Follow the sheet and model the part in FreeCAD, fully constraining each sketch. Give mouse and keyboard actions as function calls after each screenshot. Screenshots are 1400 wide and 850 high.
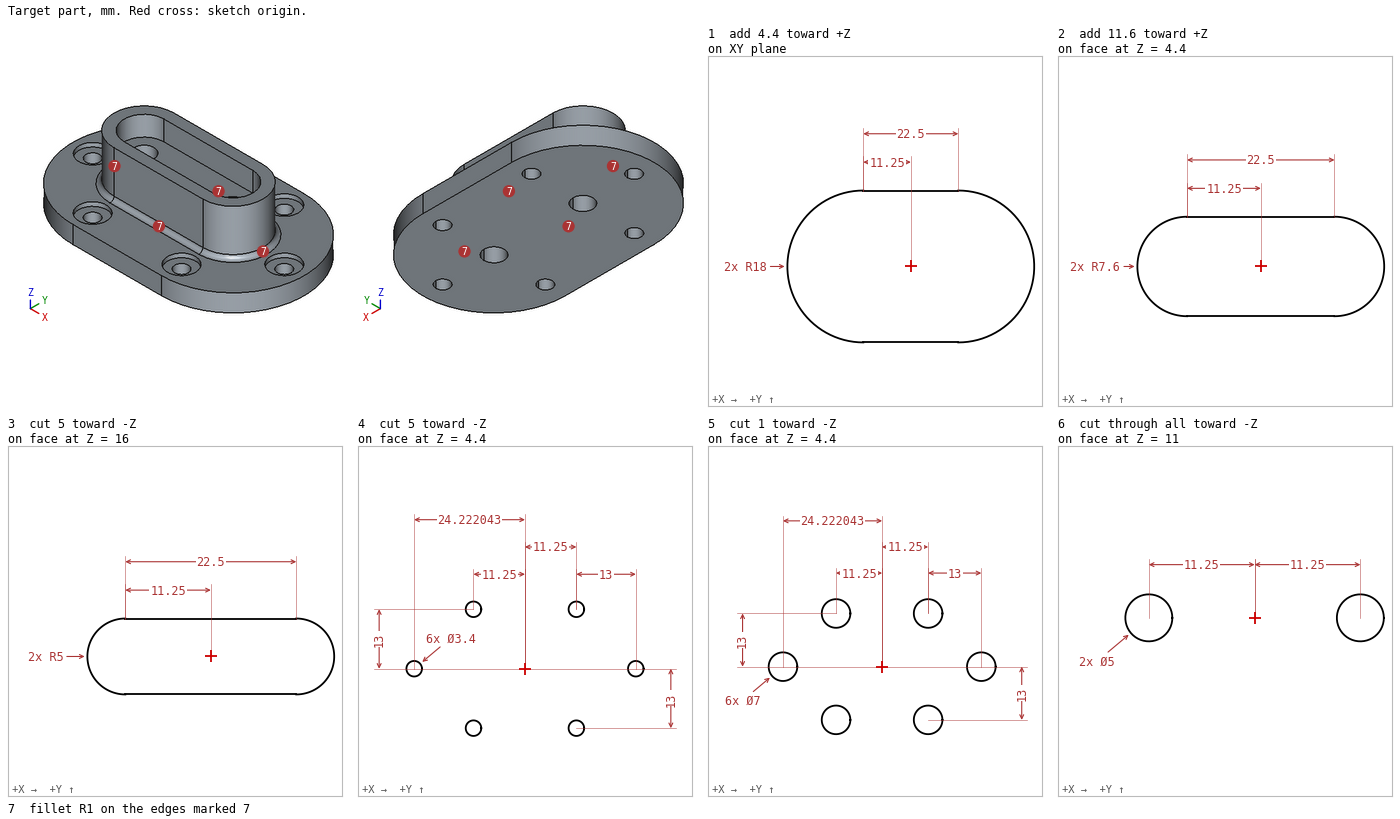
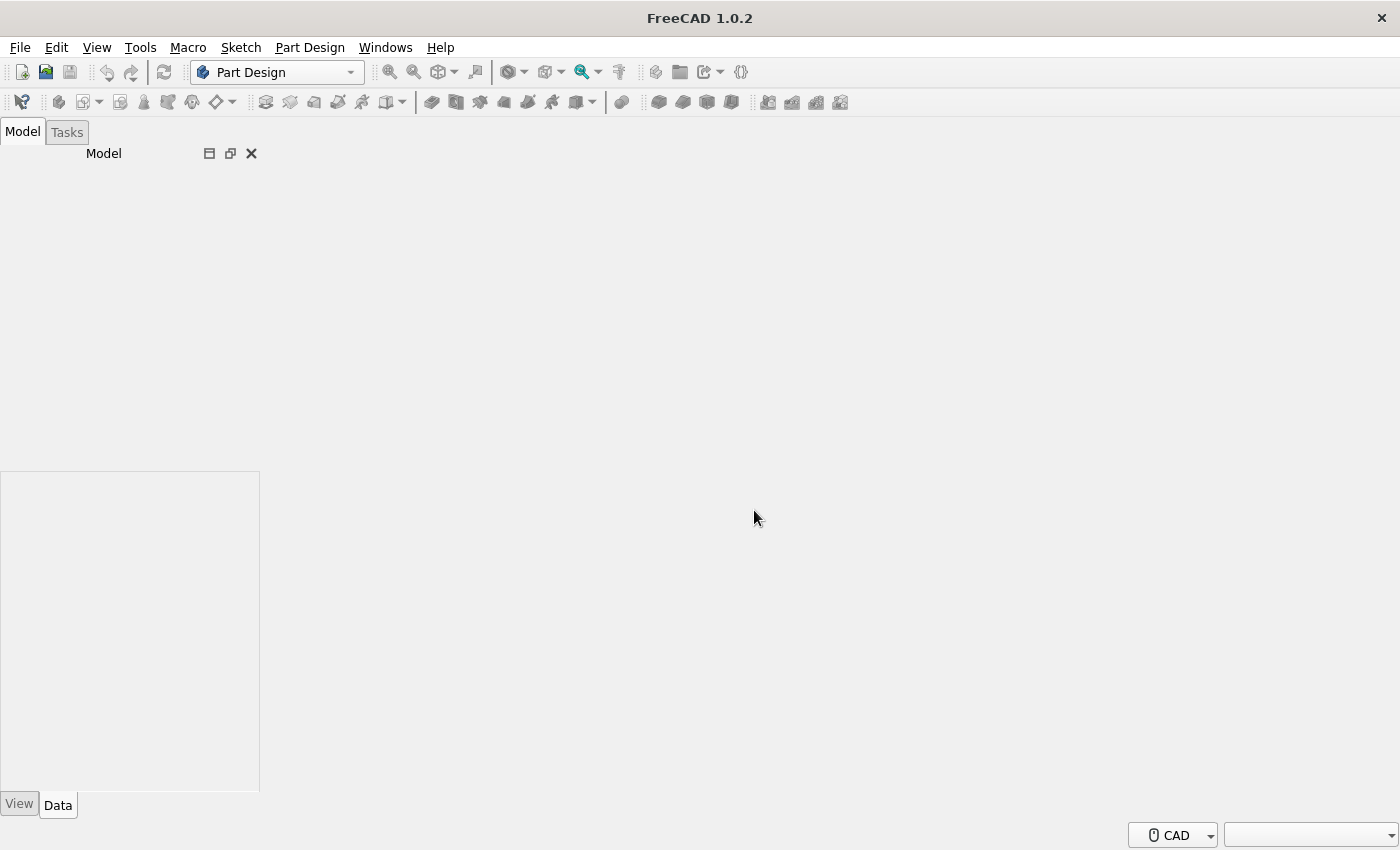
click(22, 72)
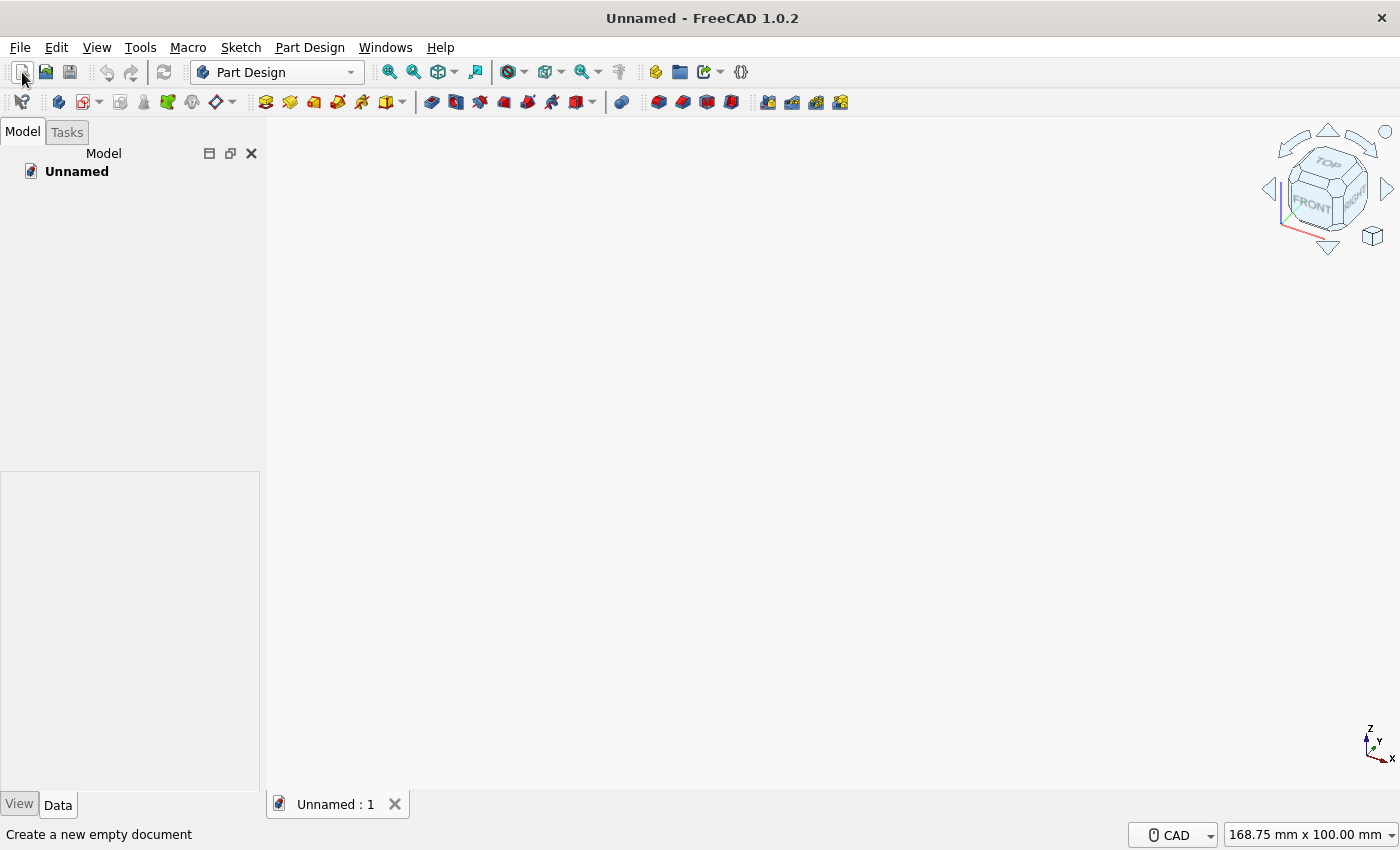
click(84, 102)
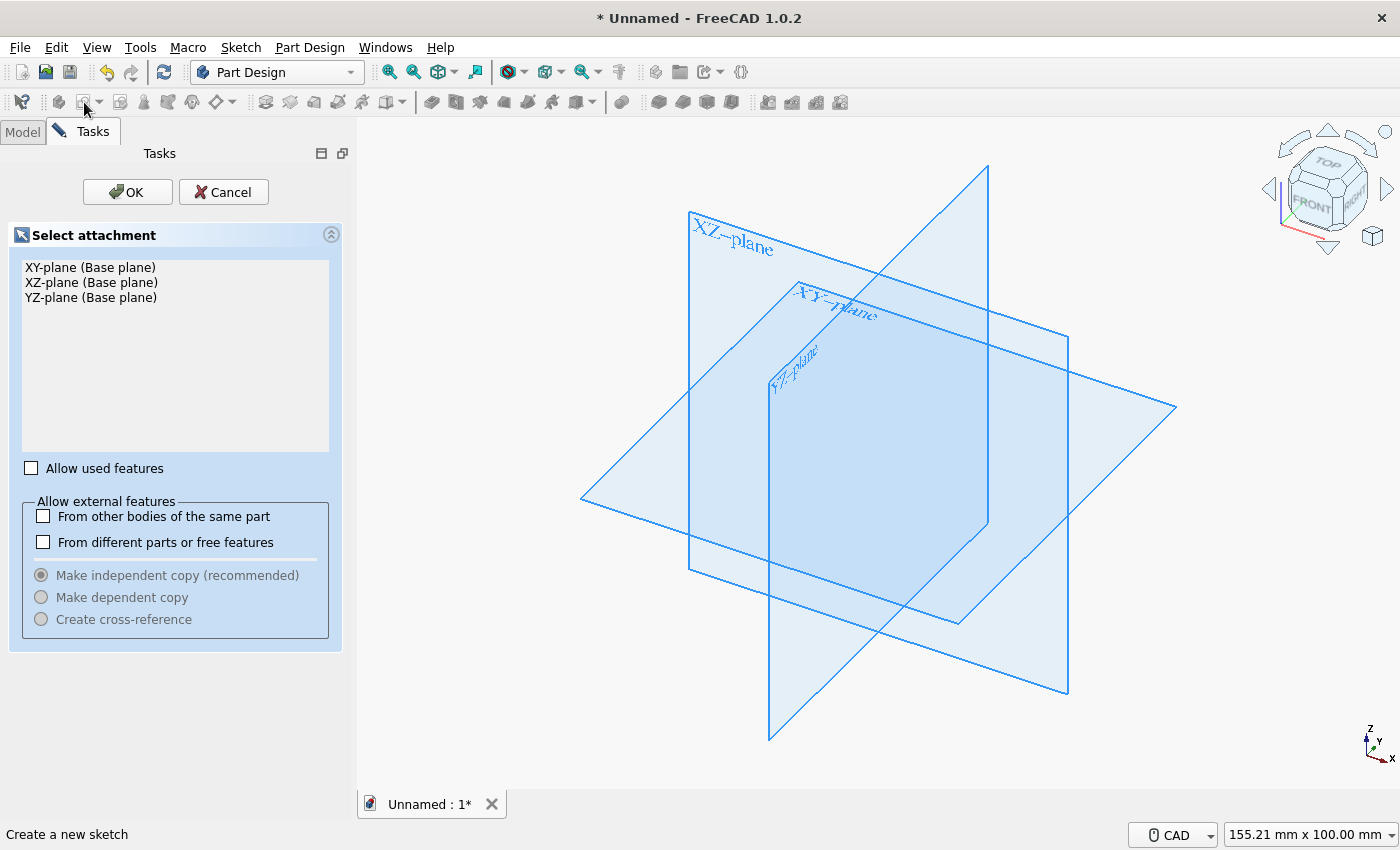
click(82, 268)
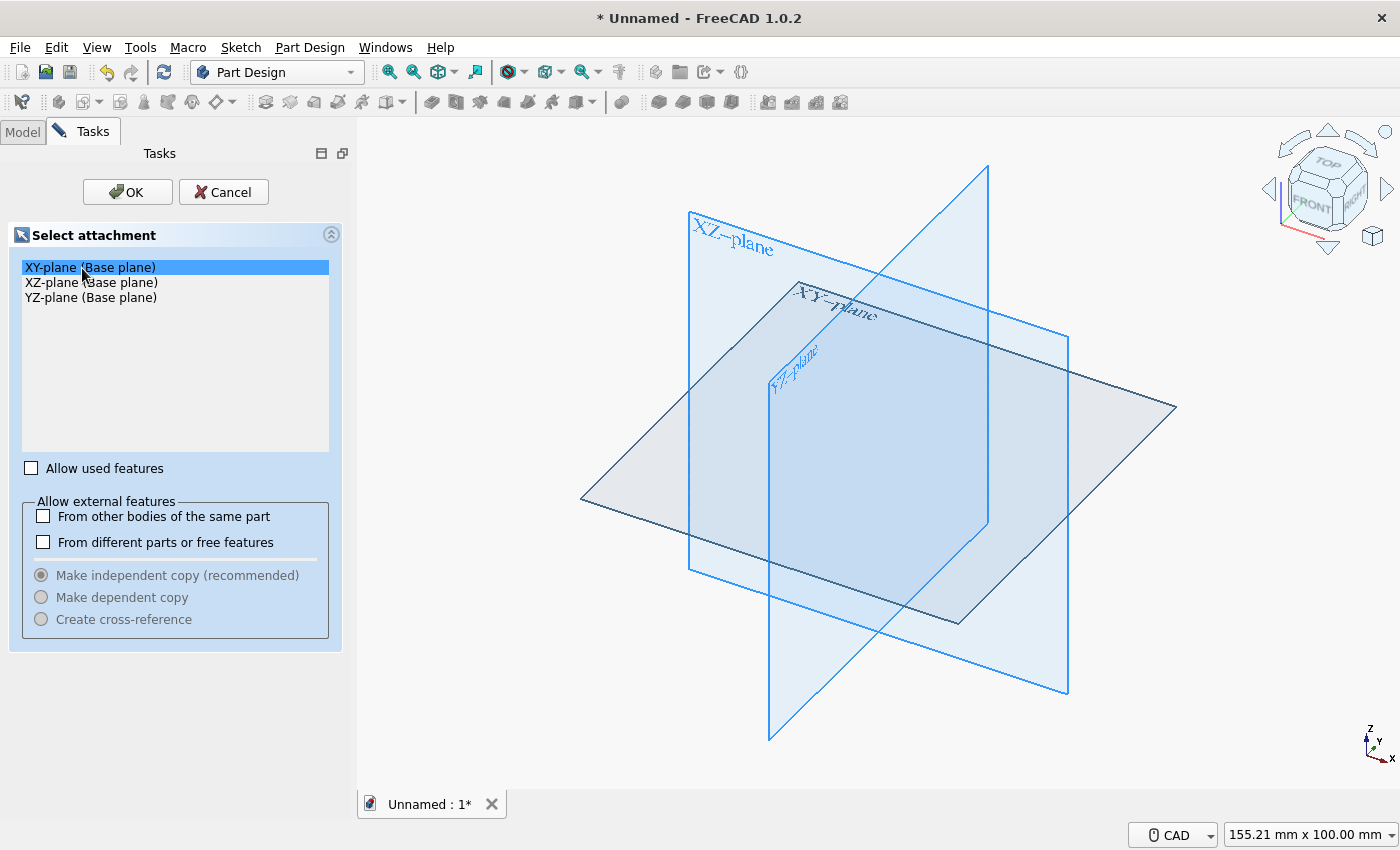
click(128, 192)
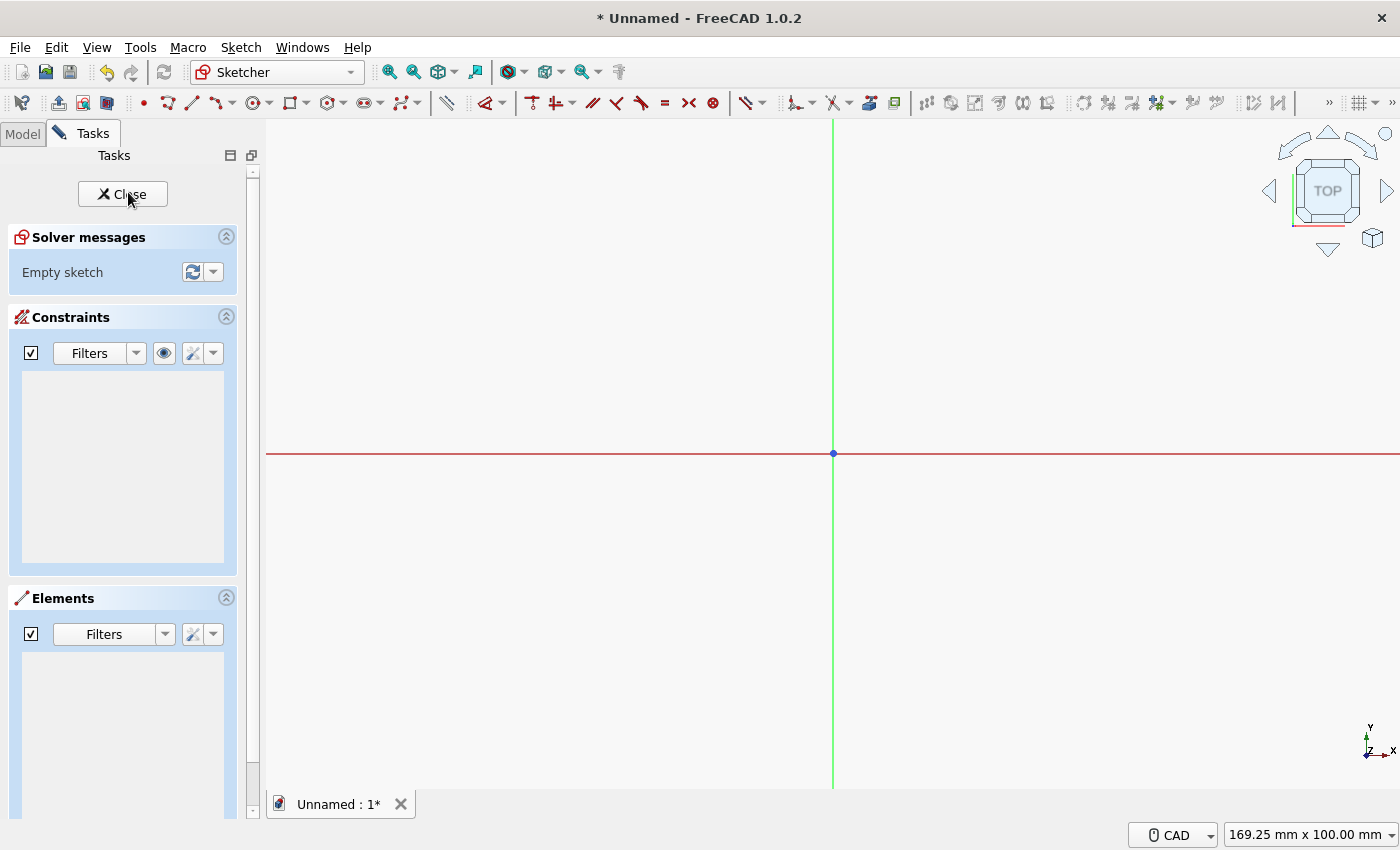
scroll(916, 454, up, 3)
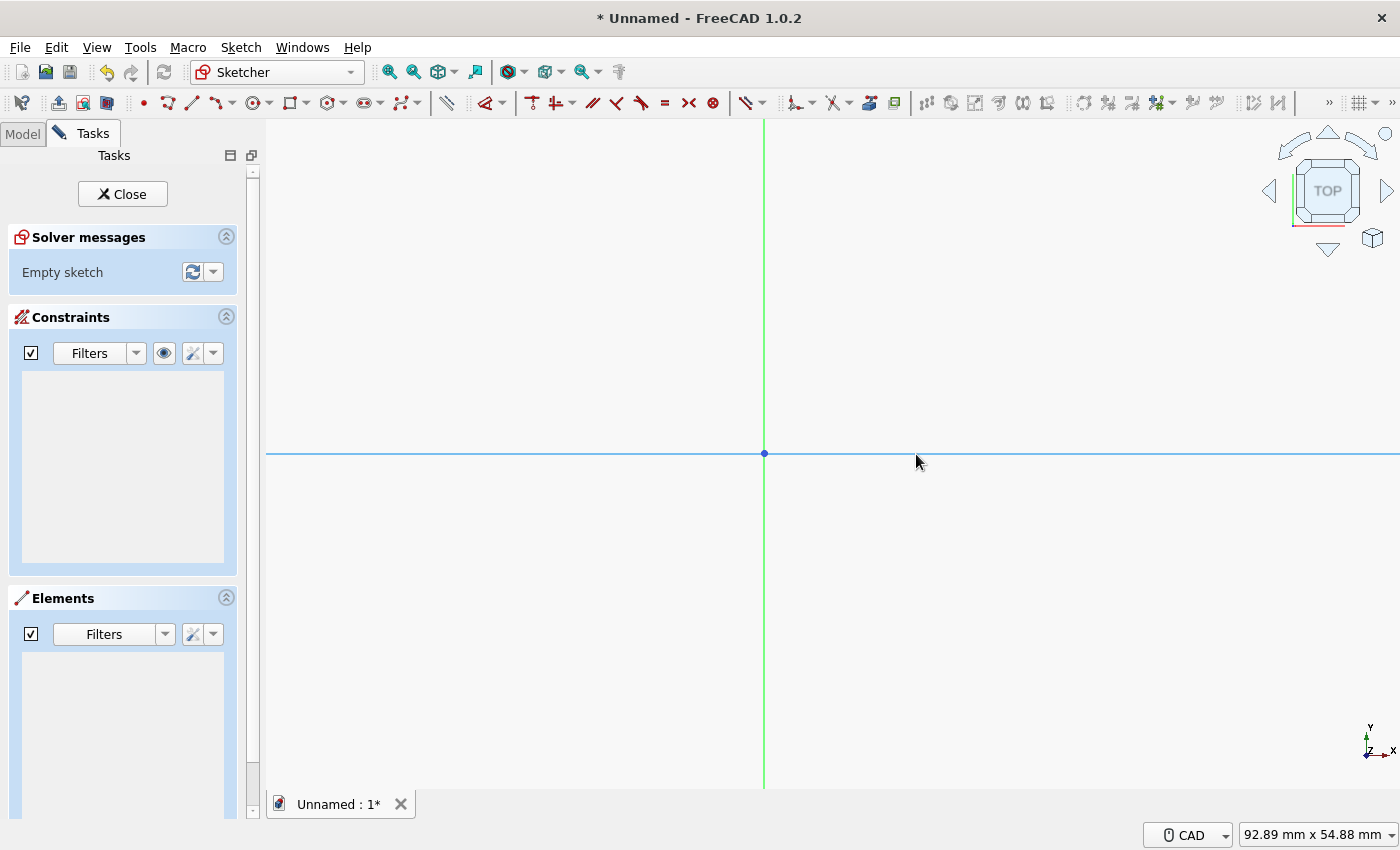
click(364, 104)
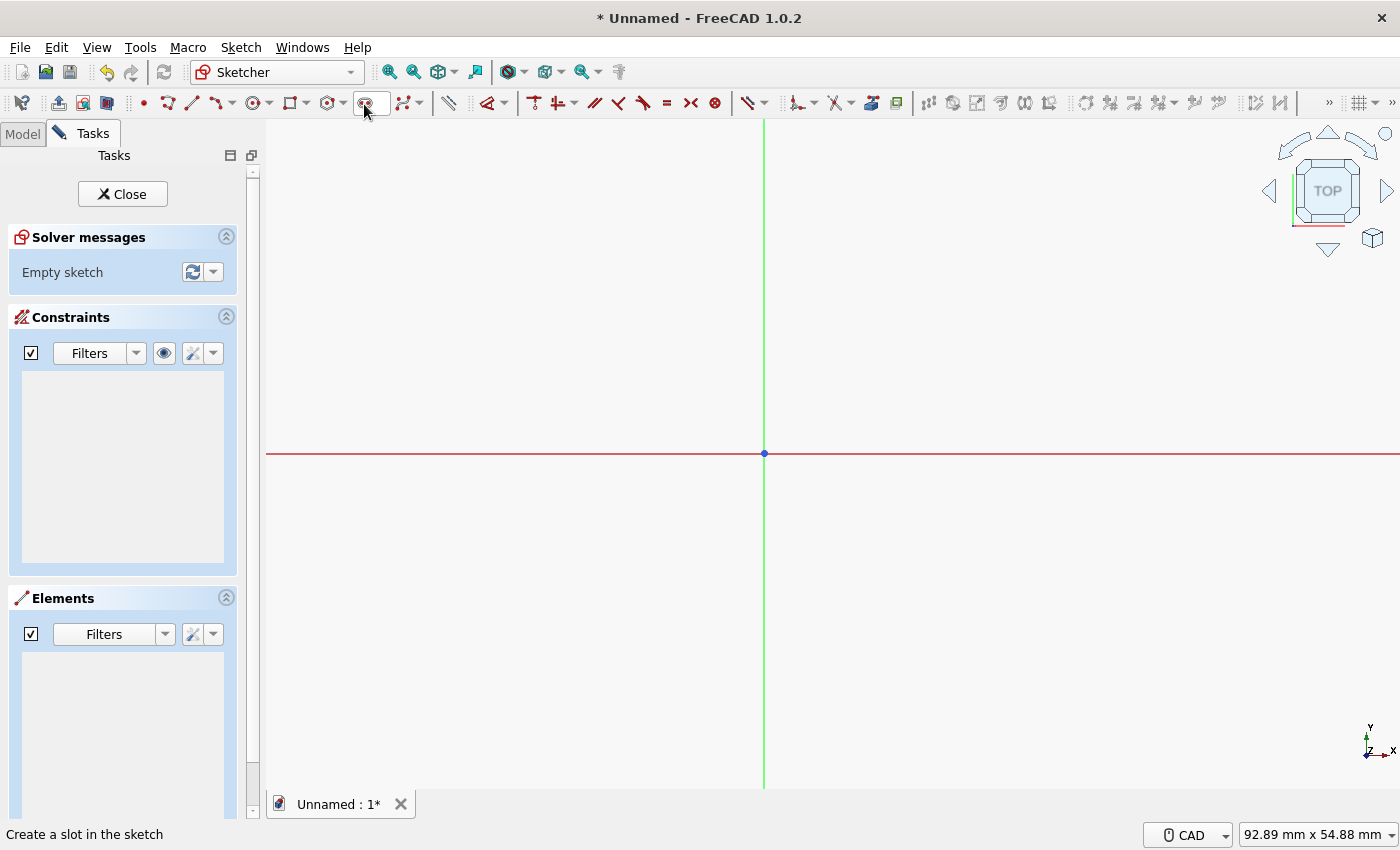
click(627, 454)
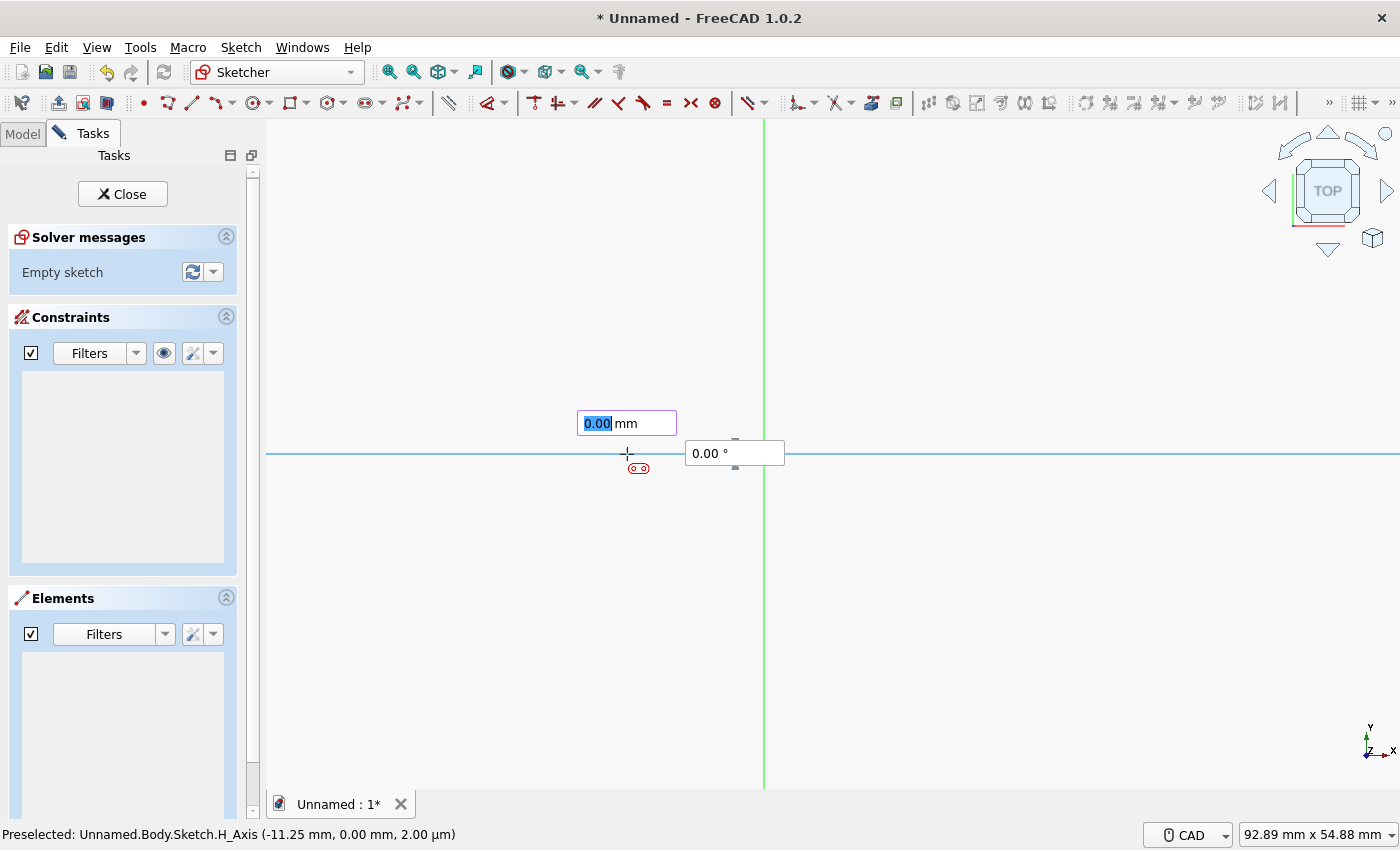
click(902, 445)